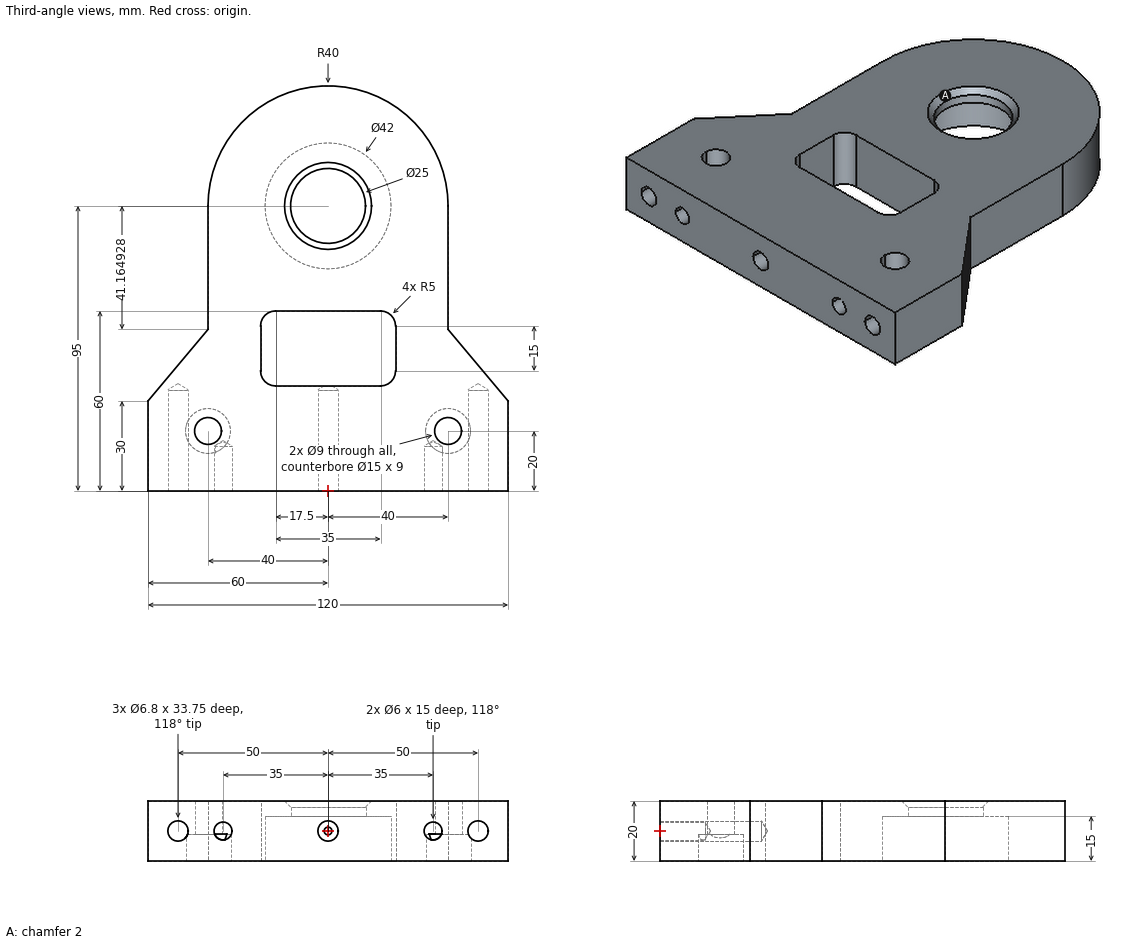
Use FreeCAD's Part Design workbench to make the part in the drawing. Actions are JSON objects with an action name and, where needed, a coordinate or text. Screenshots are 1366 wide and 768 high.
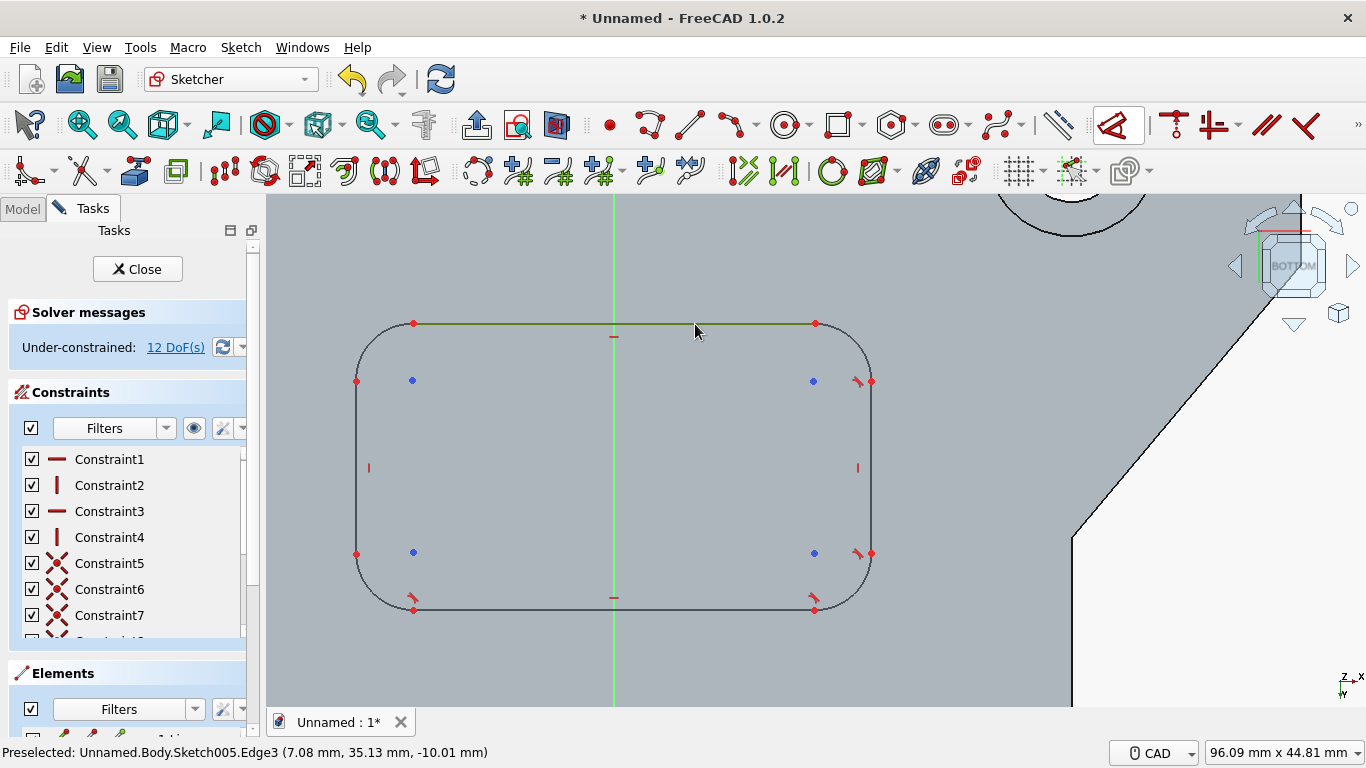
{"action": "left_click", "coordinate": [865, 356]}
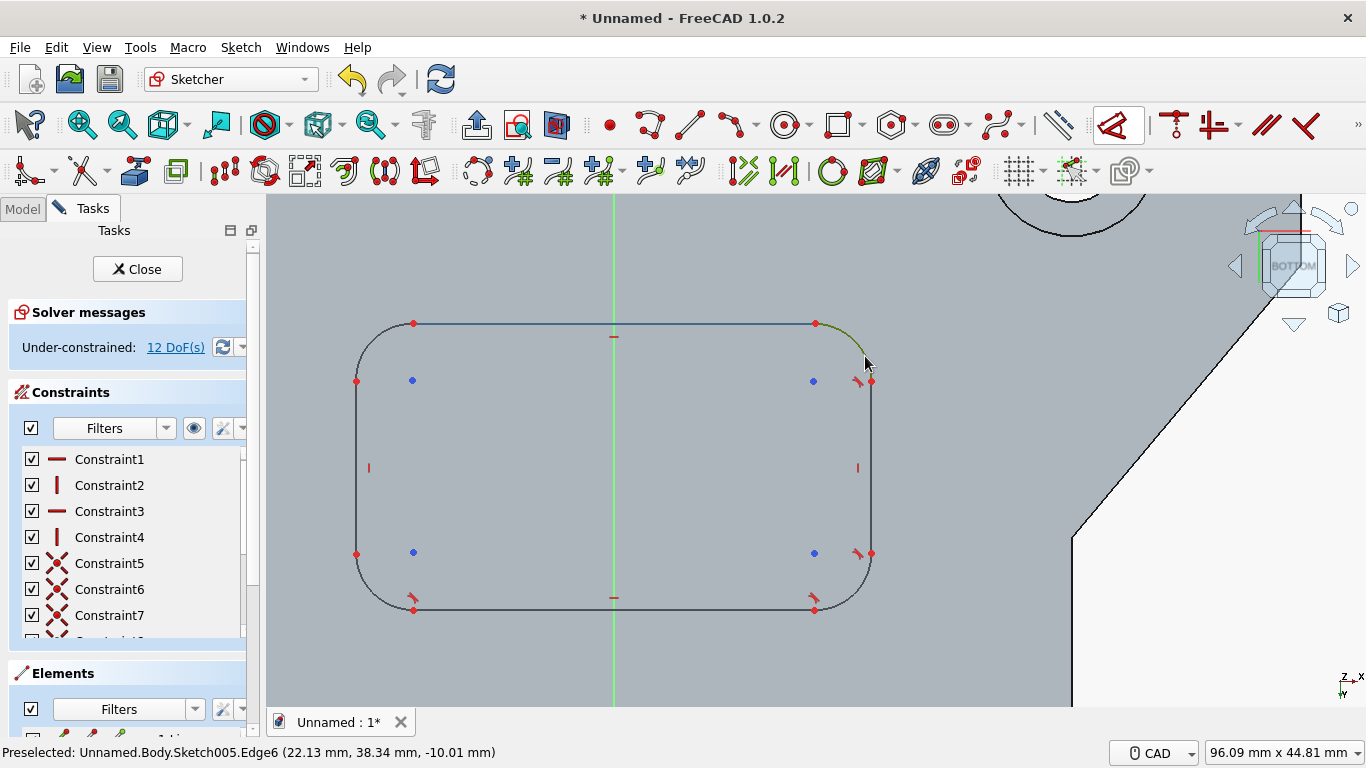
{"action": "key", "text": "t"}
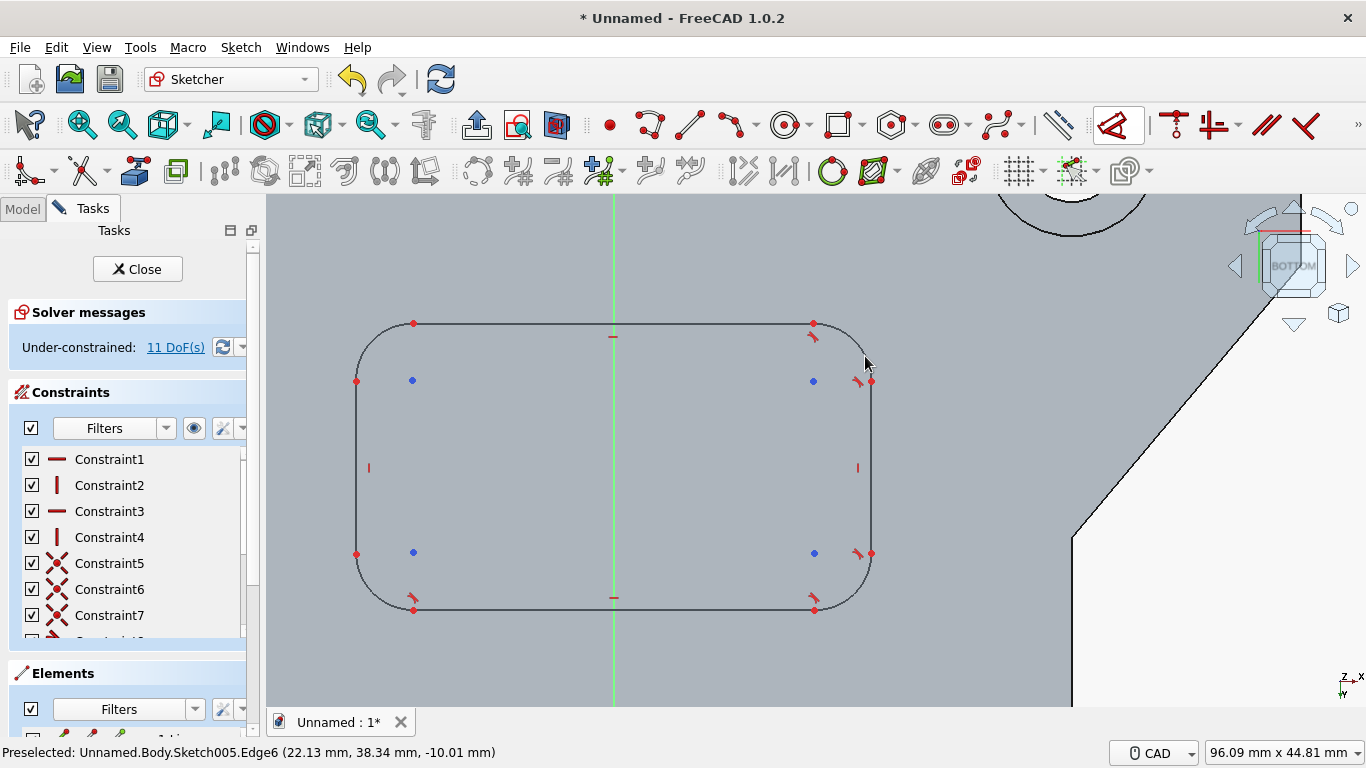
{"action": "left_click", "coordinate": [694, 324]}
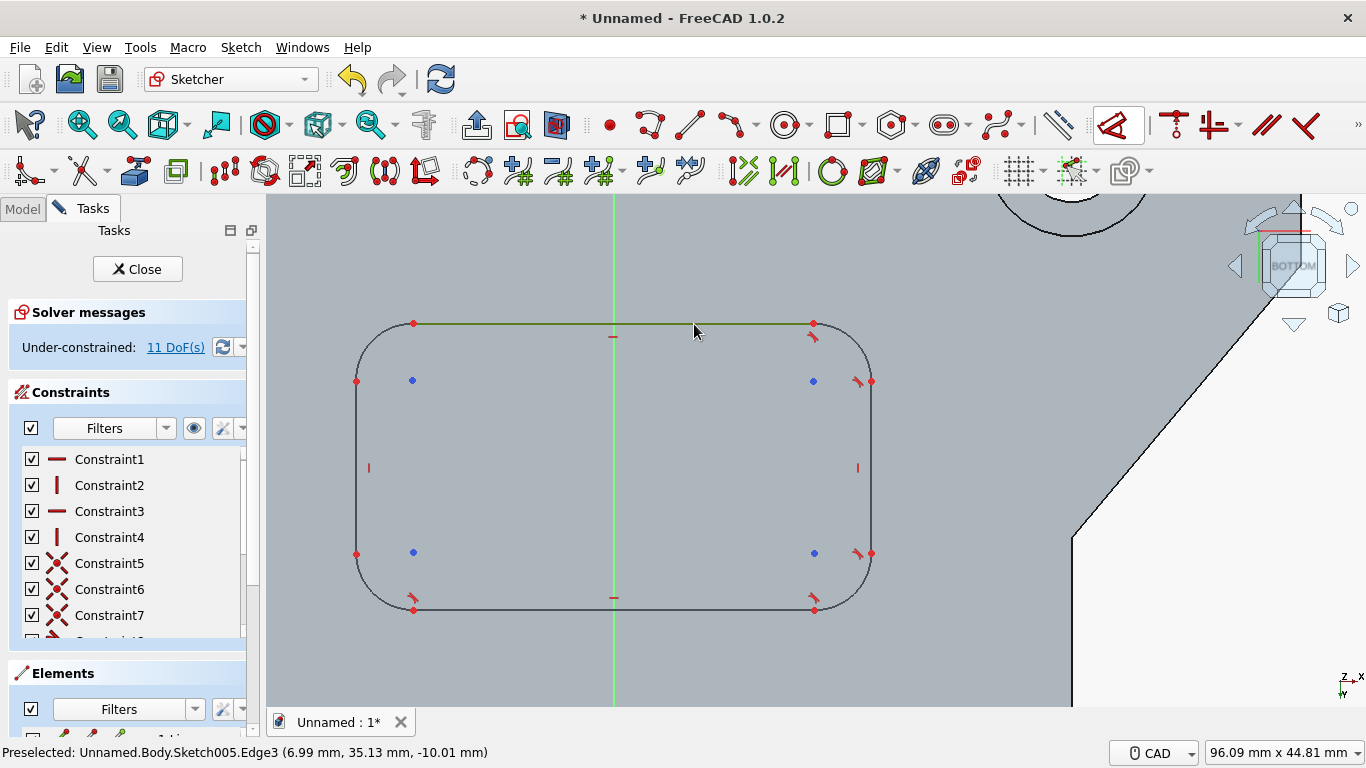
{"action": "left_click", "coordinate": [387, 330]}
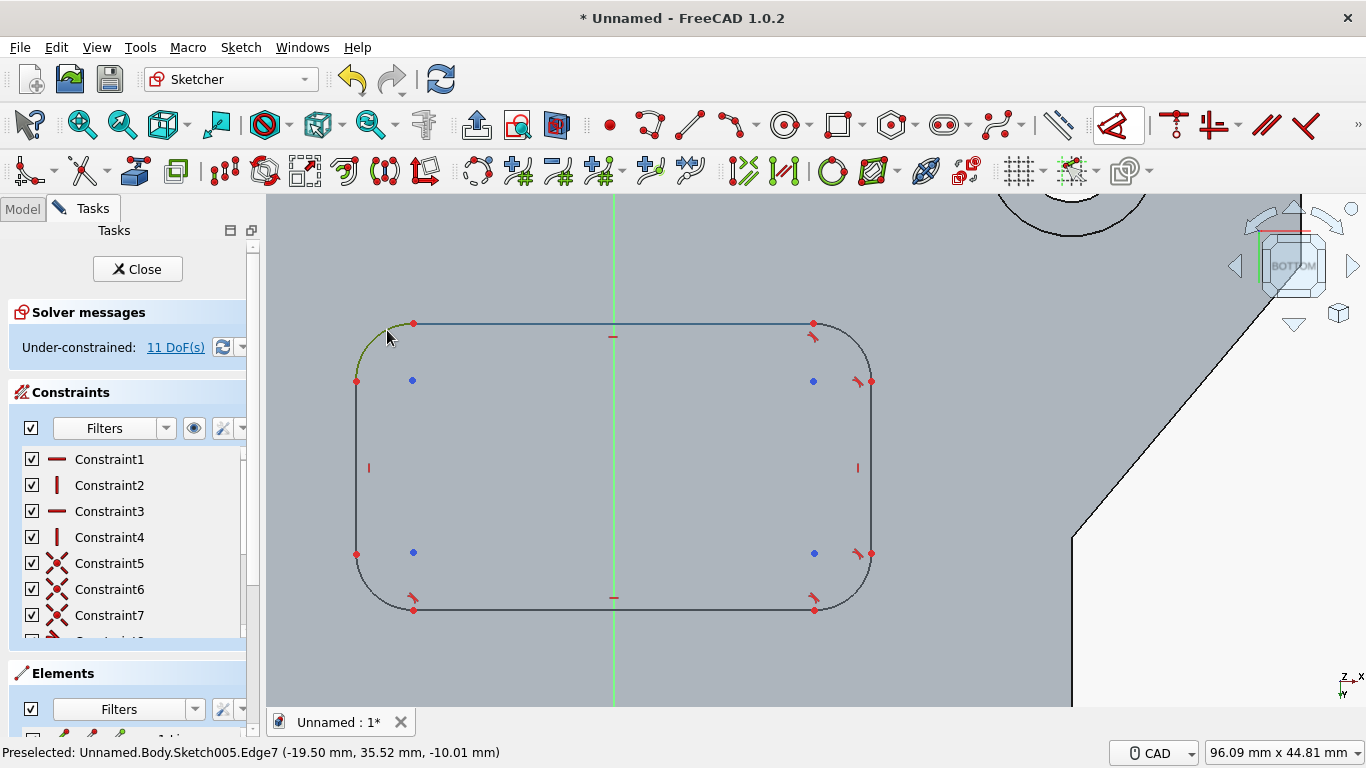
{"action": "key", "text": "t"}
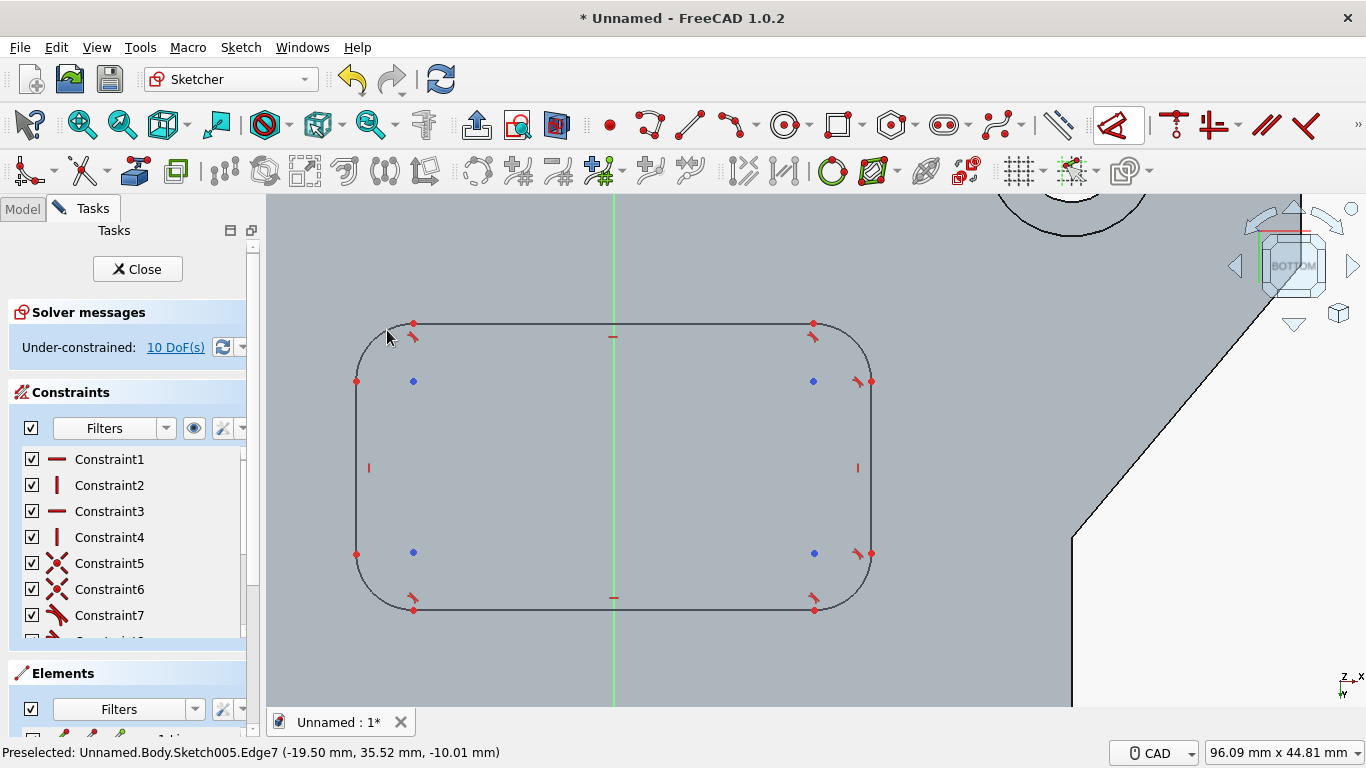
{"action": "left_click", "coordinate": [356, 433]}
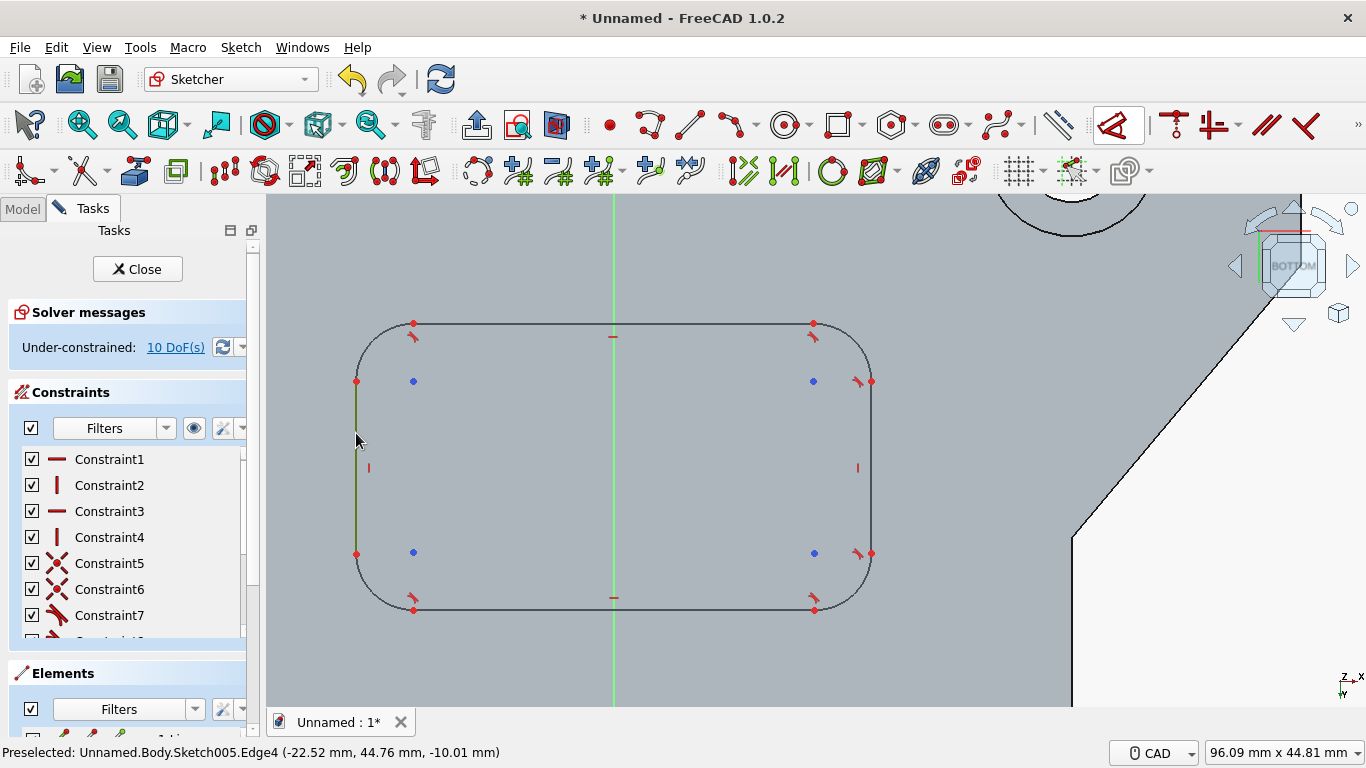
{"action": "left_click", "coordinate": [388, 330]}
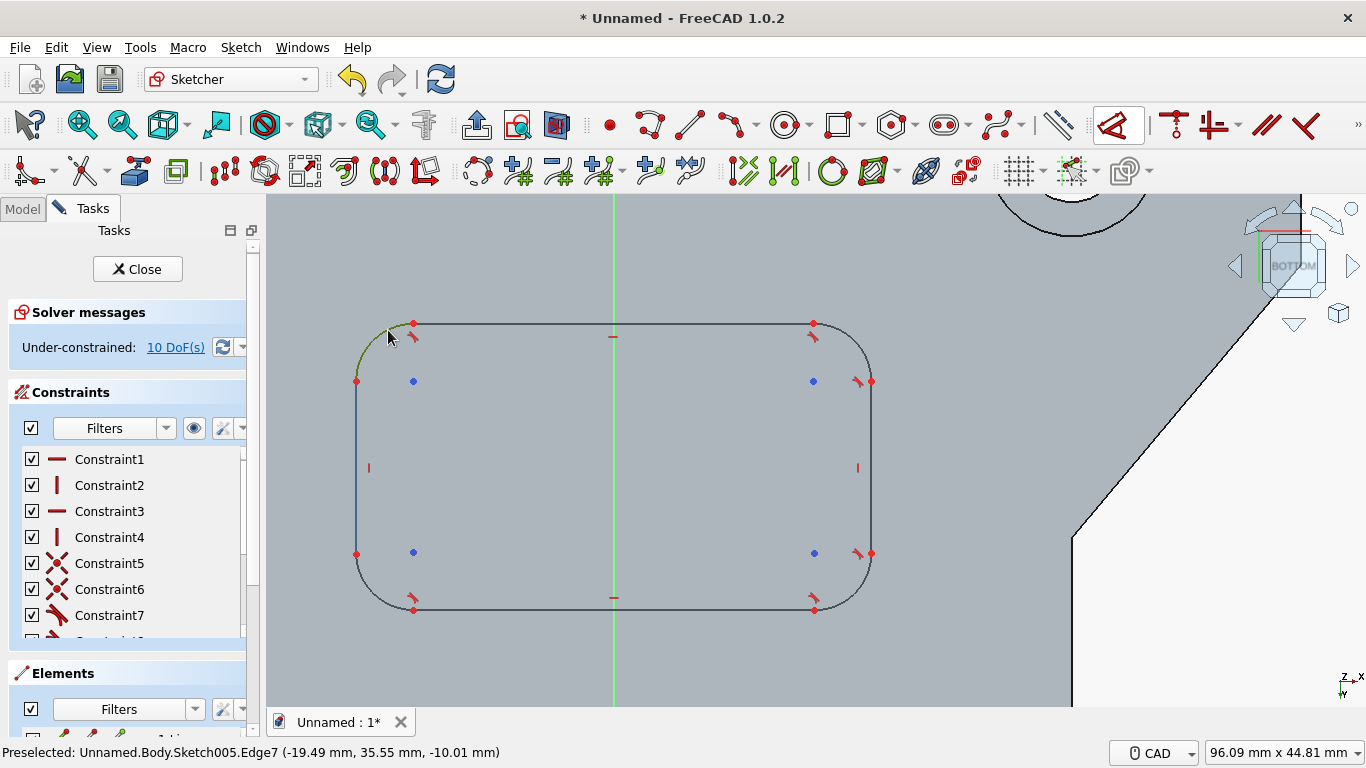
{"action": "key", "text": "t"}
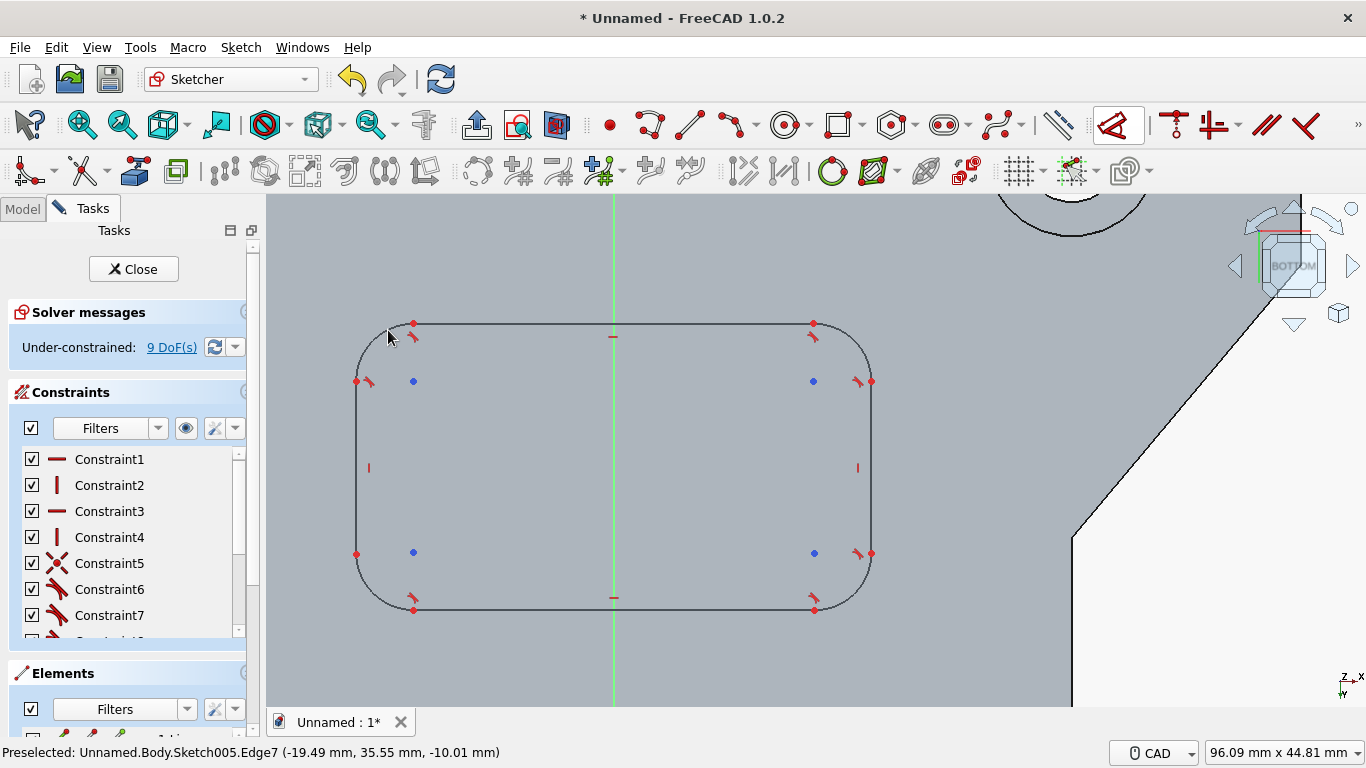
{"action": "left_click", "coordinate": [356, 433]}